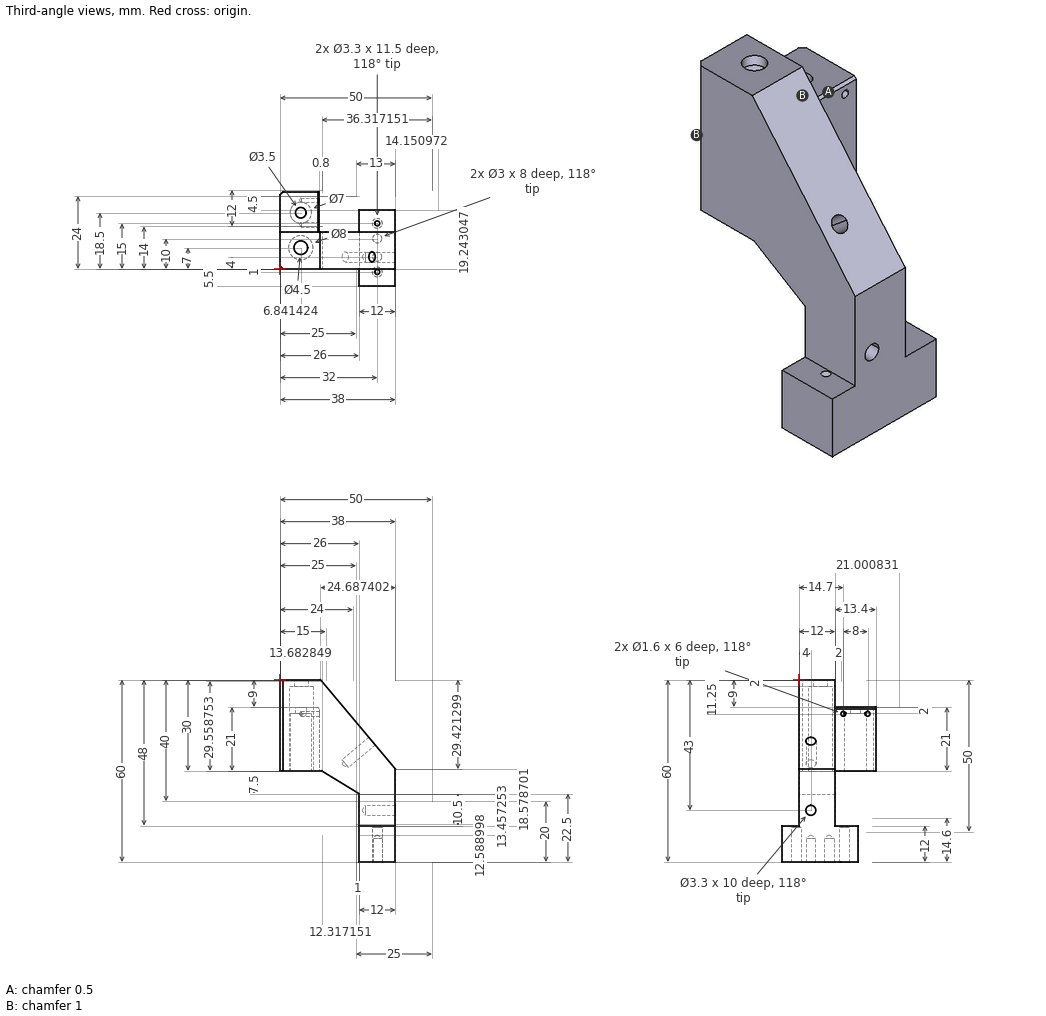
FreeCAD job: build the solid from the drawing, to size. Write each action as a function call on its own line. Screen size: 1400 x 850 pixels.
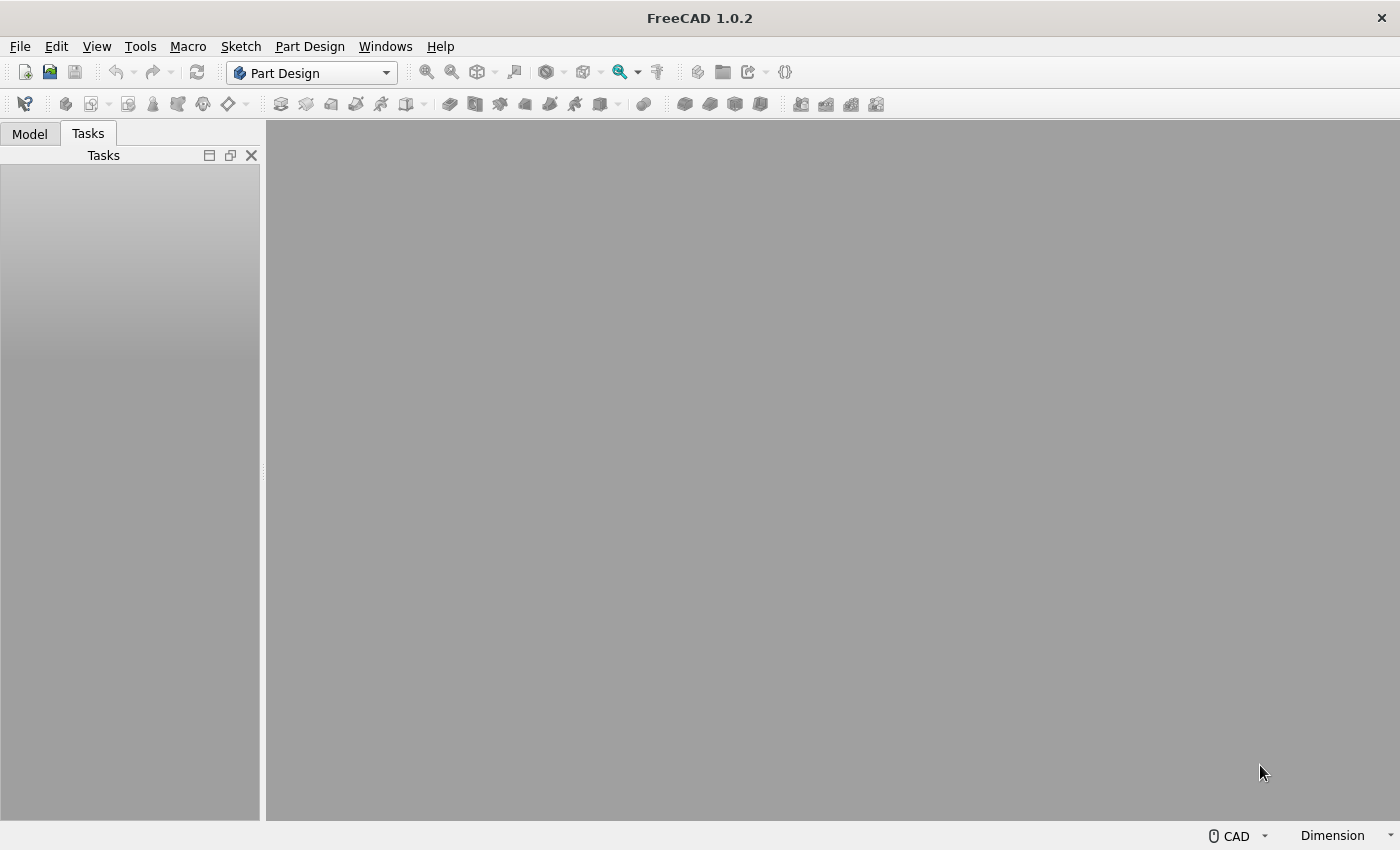
key(ctrl+n)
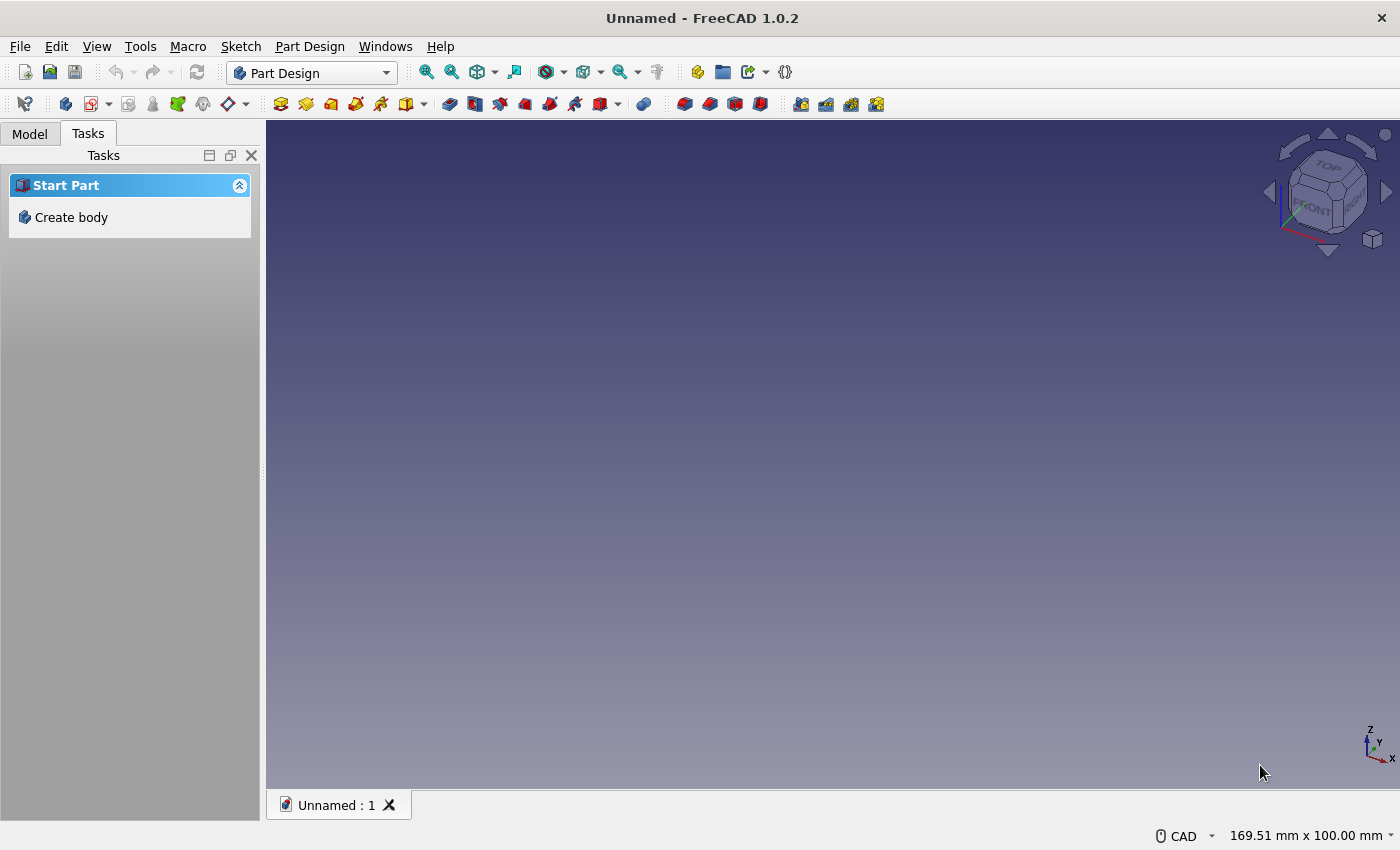
click(90, 104)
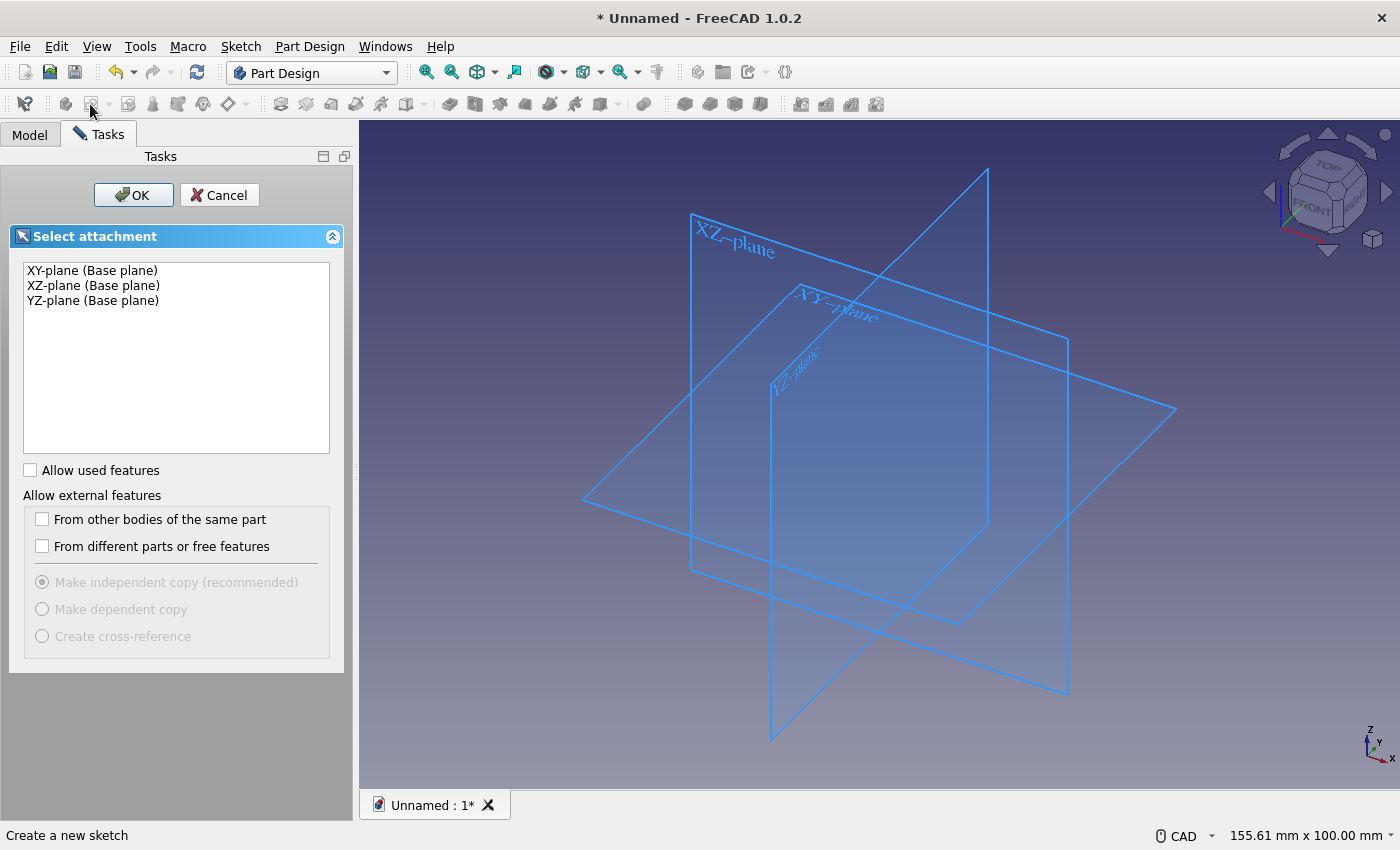
click(84, 286)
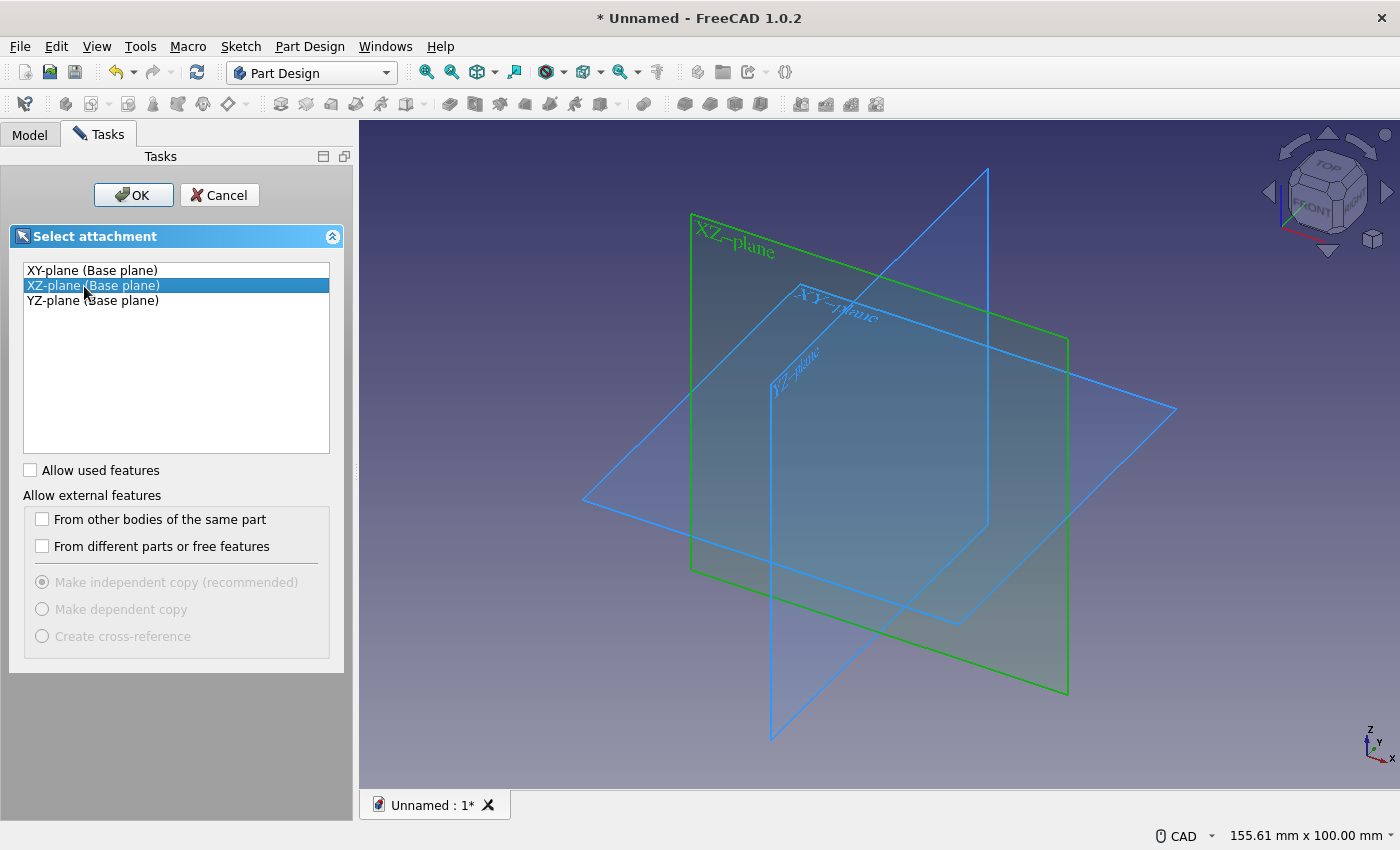
click(134, 195)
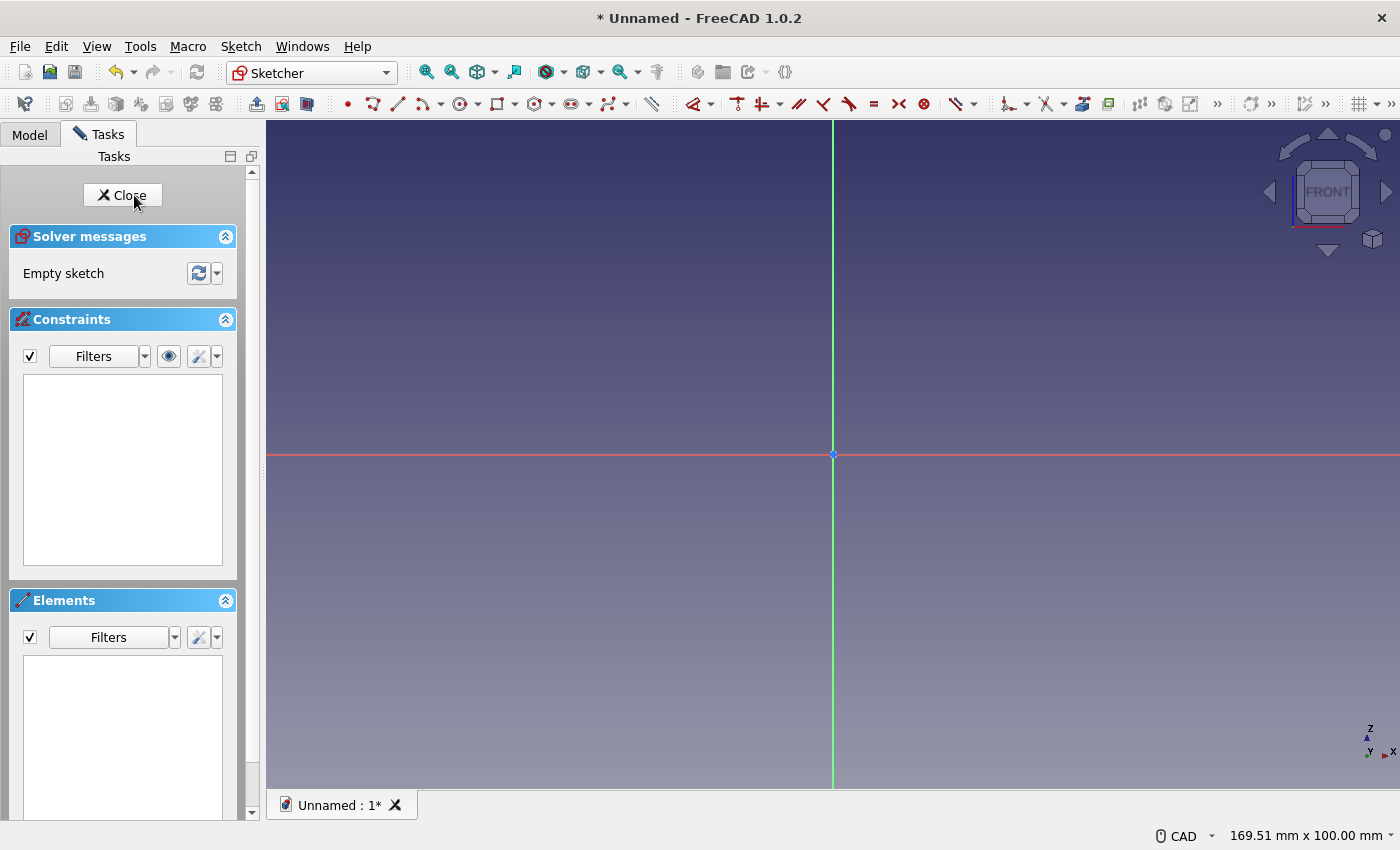
scroll(294, 148, down, 1)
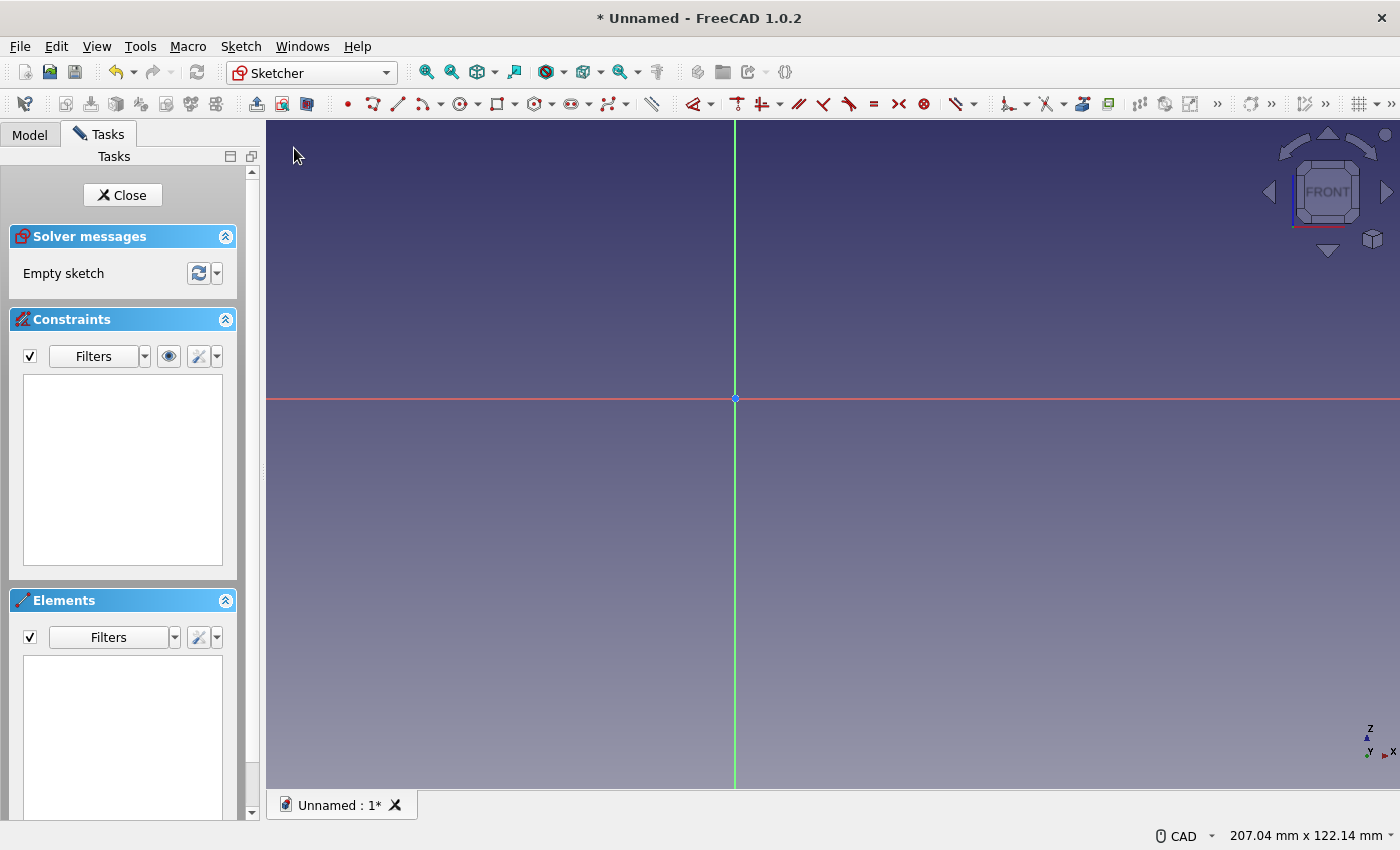
click(373, 104)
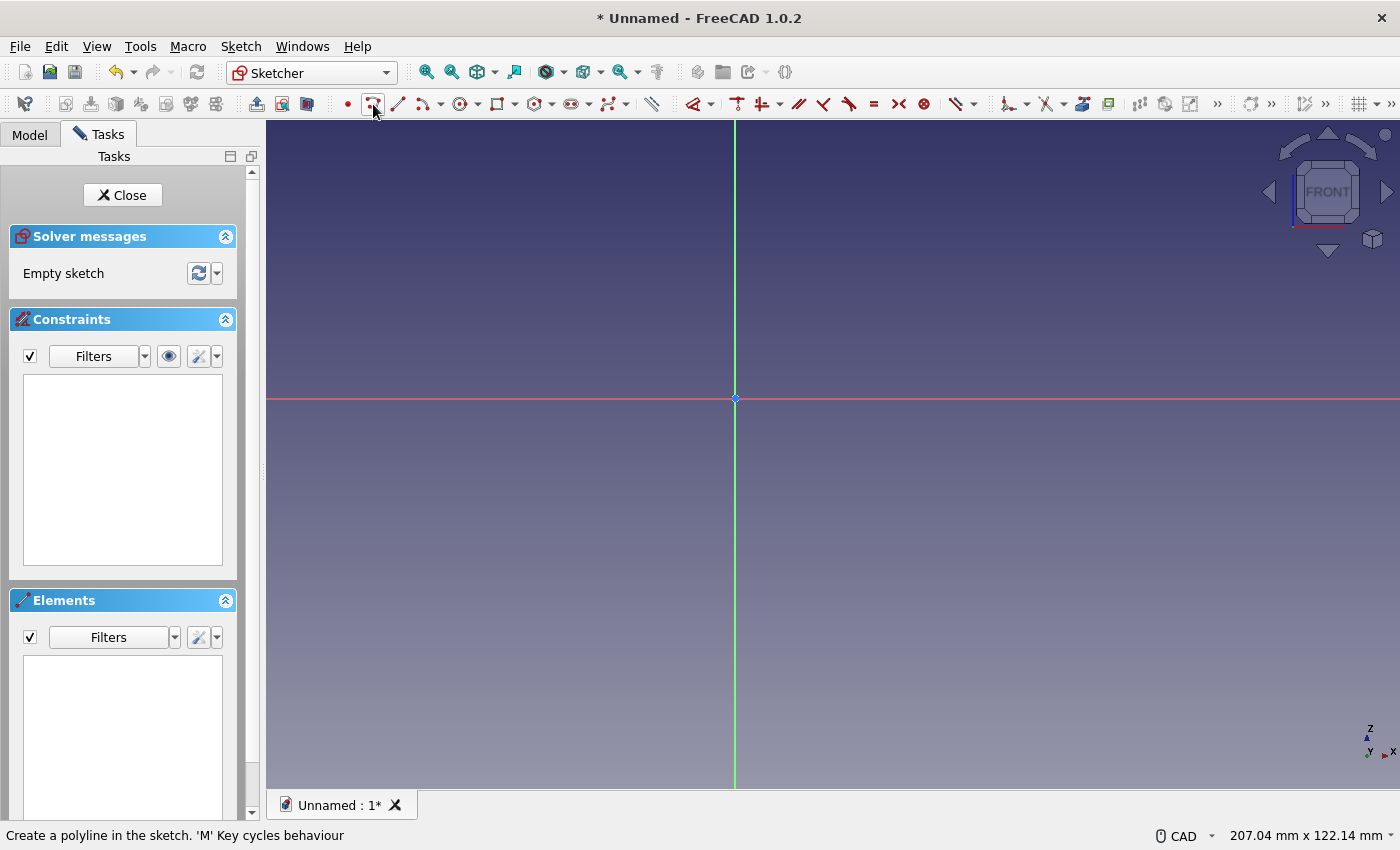
click(735, 399)
click(867, 408)
click(1009, 618)
click(1009, 728)
click(872, 728)
click(872, 659)
click(810, 563)
click(744, 563)
click(735, 399)
key(Escape)
key(Escape)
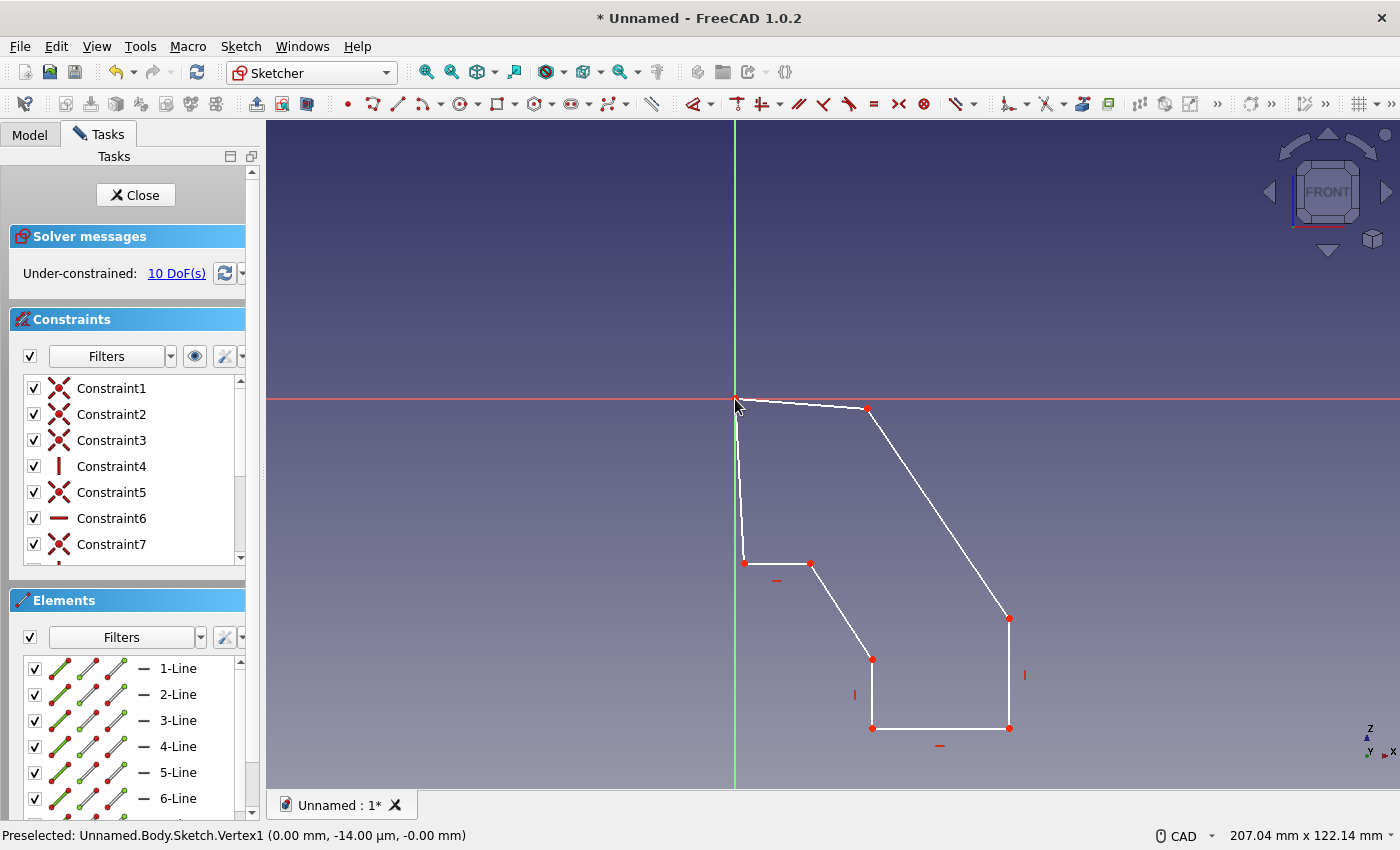
click(775, 402)